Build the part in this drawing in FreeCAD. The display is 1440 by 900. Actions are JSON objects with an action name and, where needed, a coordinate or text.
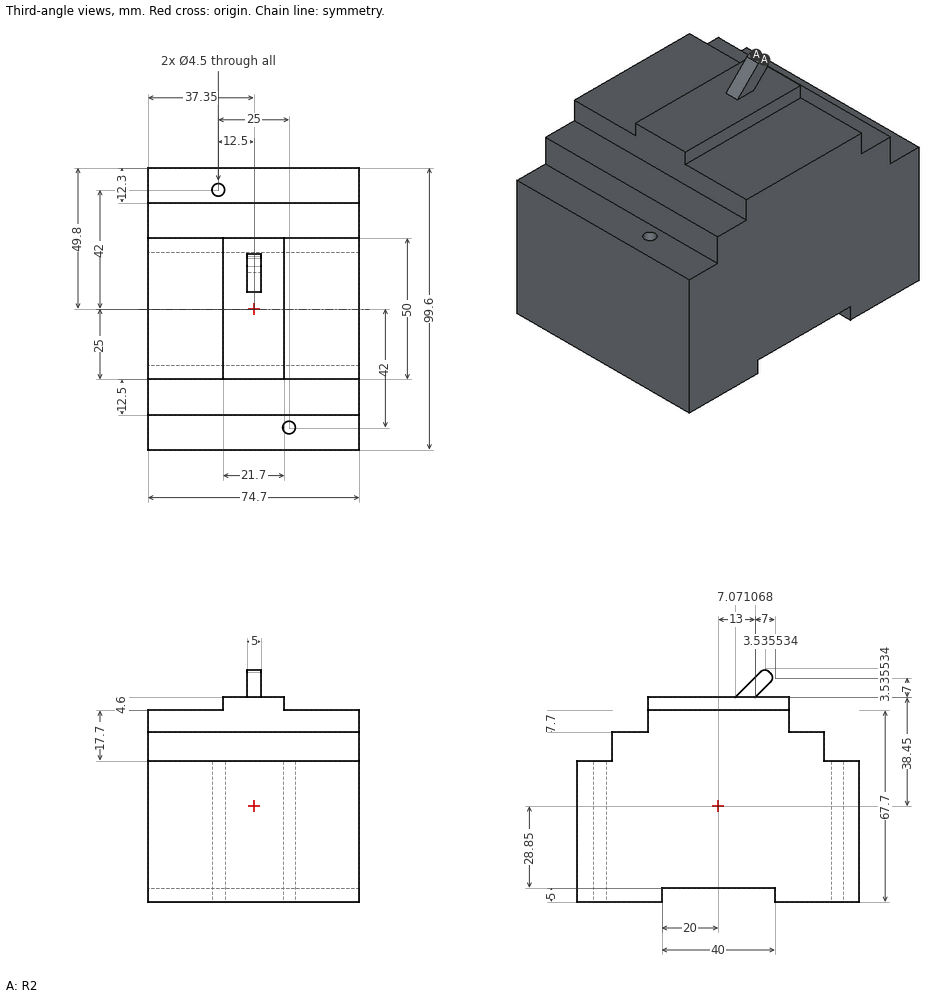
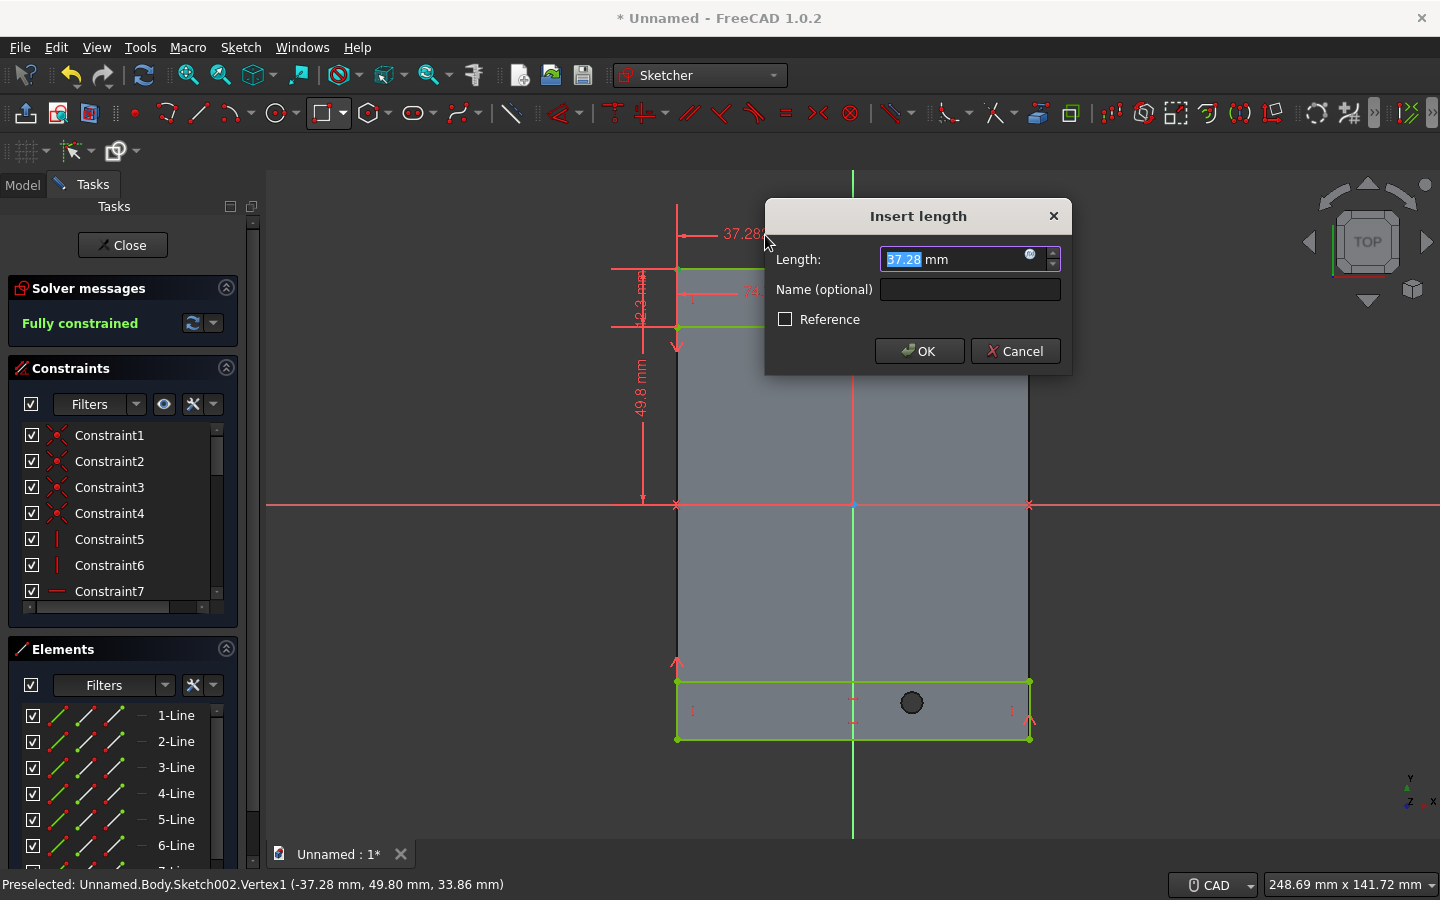
{"action": "type", "text": "37.35"}
{"action": "key", "text": "Return"}
{"action": "key", "text": "Escape"}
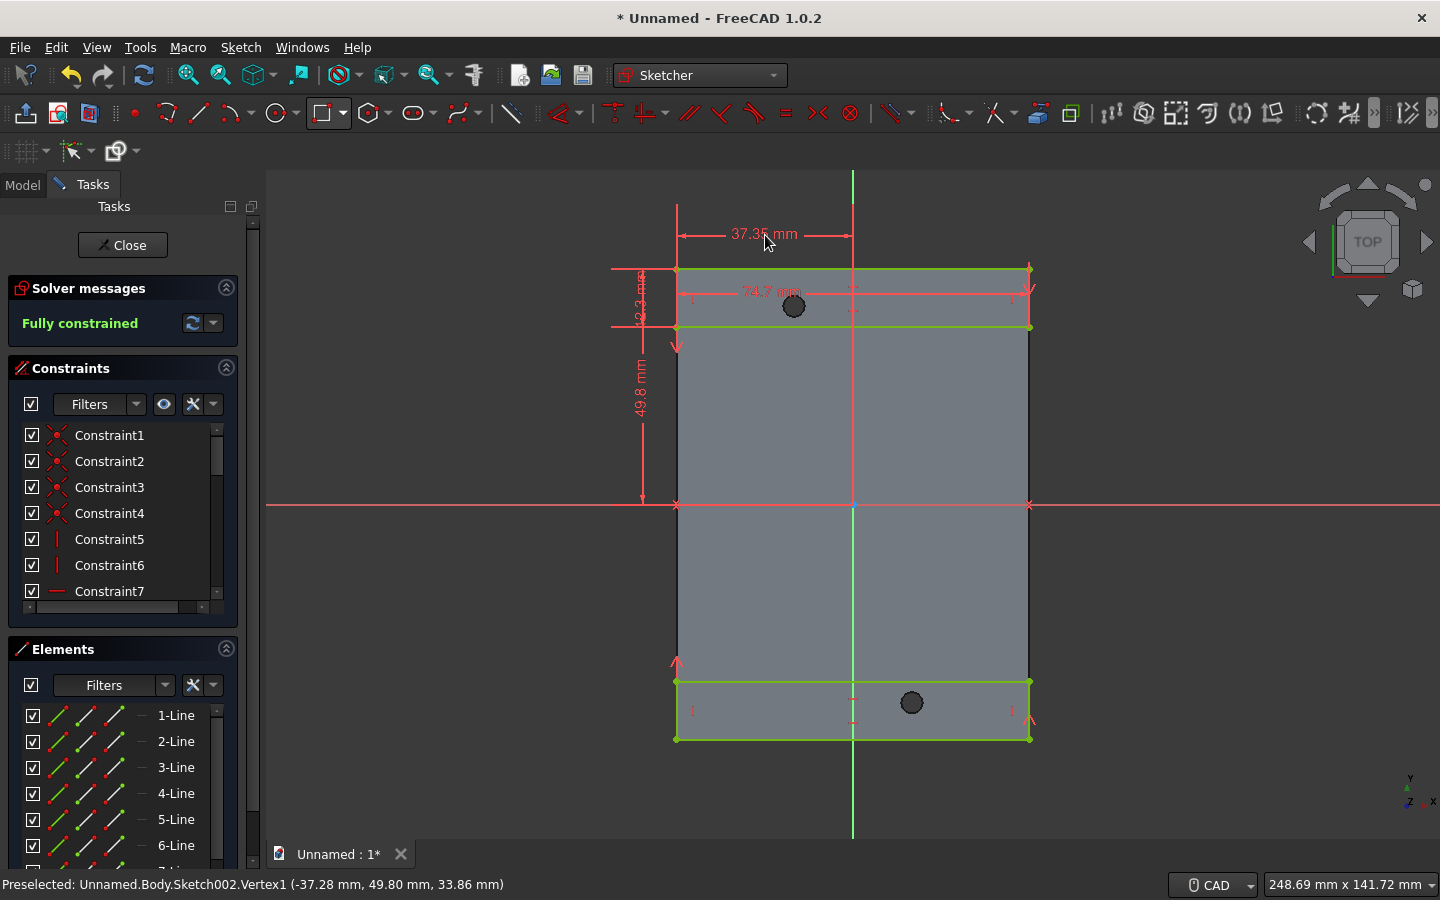
{"action": "left_click", "coordinate": [123, 245]}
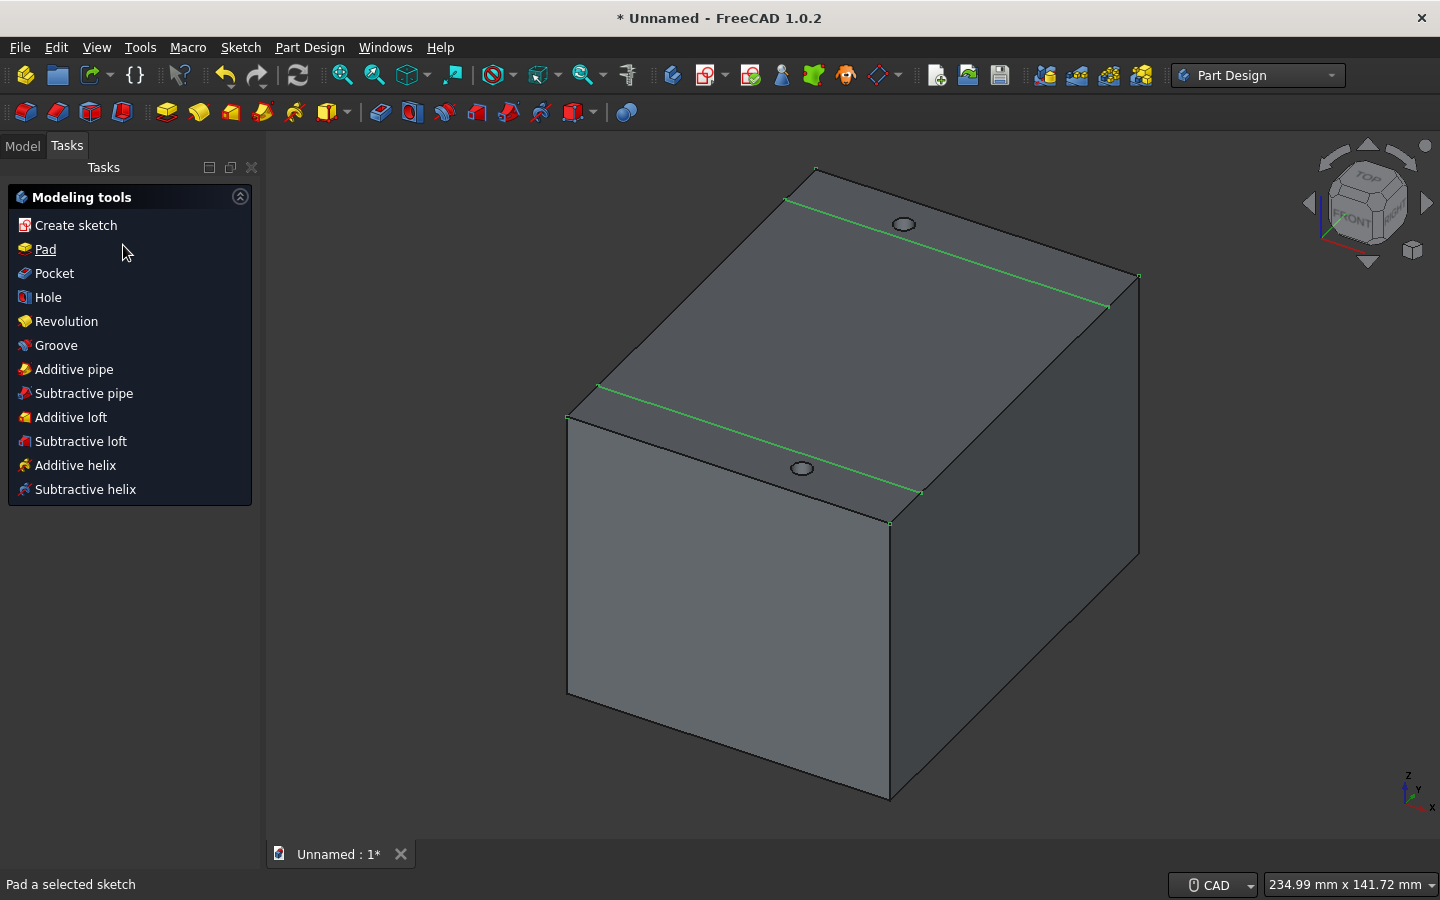
{"action": "left_click", "coordinate": [382, 112]}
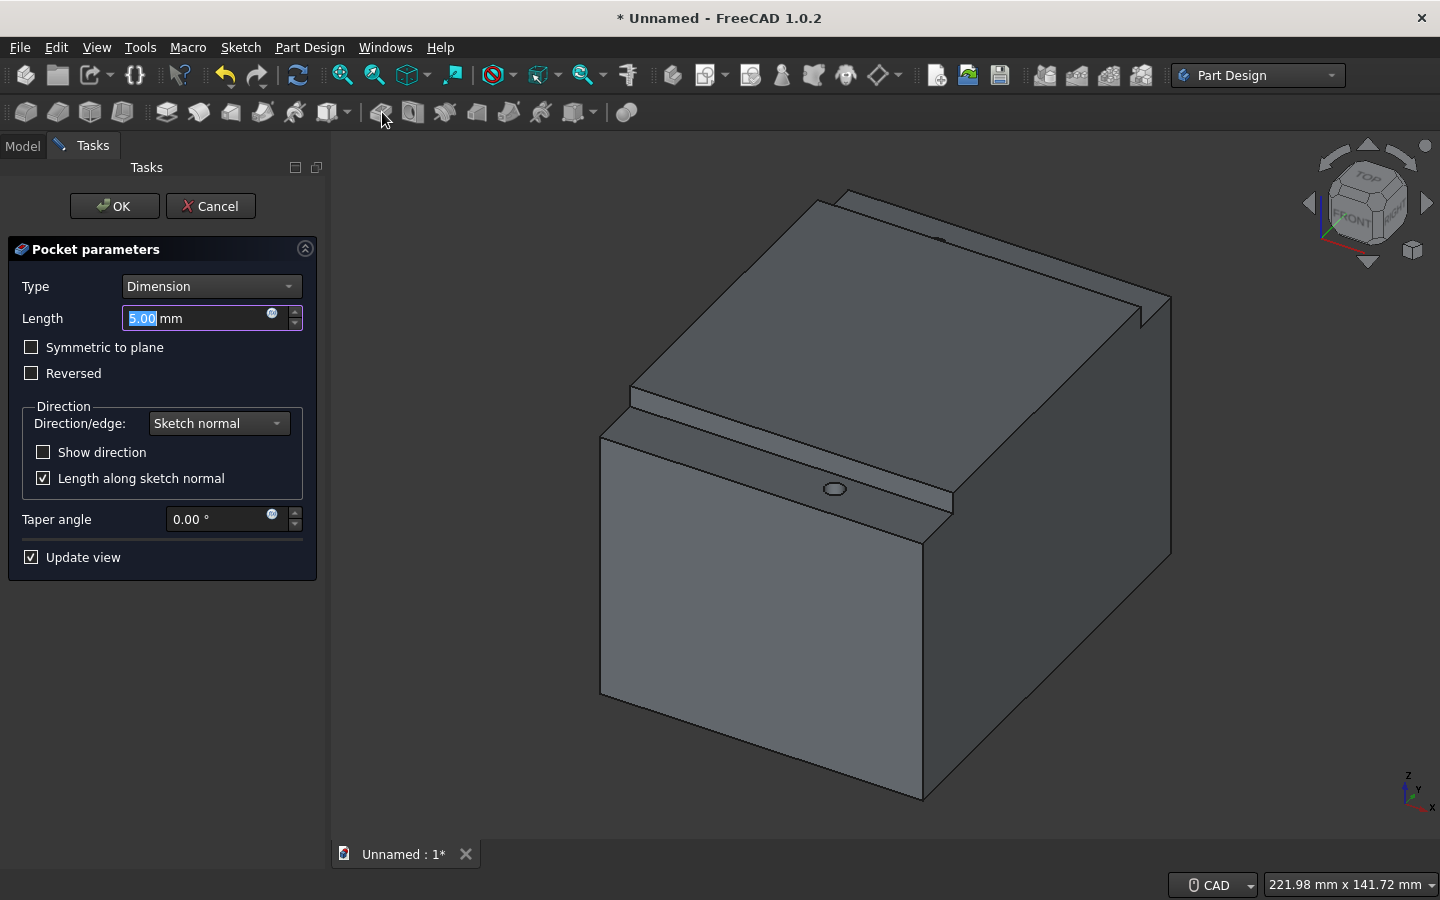
{"action": "type", "text": "17.7"}
{"action": "key", "text": "Tab"}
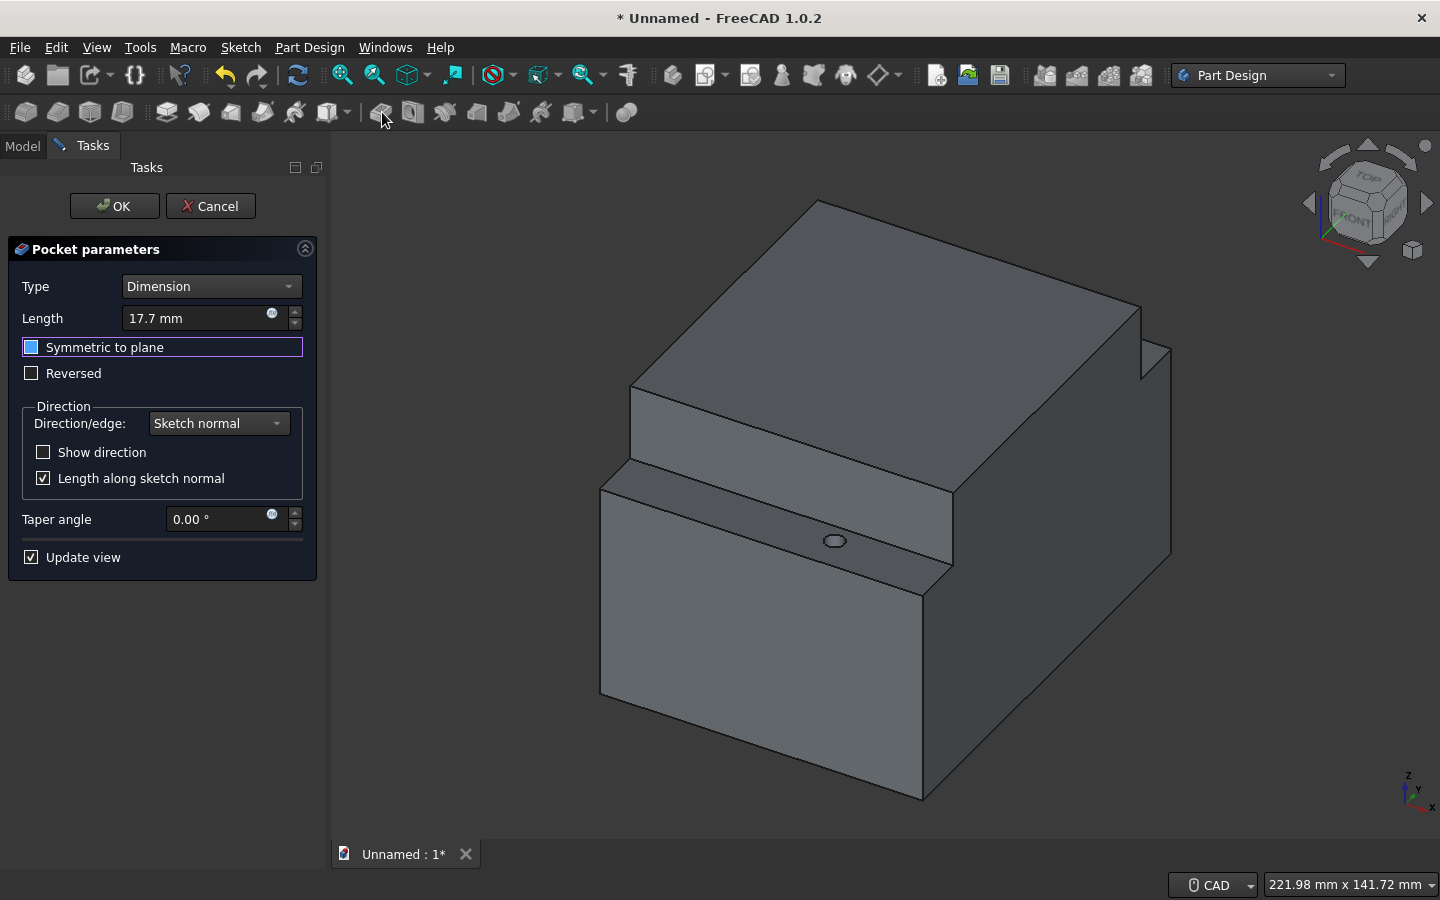
{"action": "left_click", "coordinate": [115, 206]}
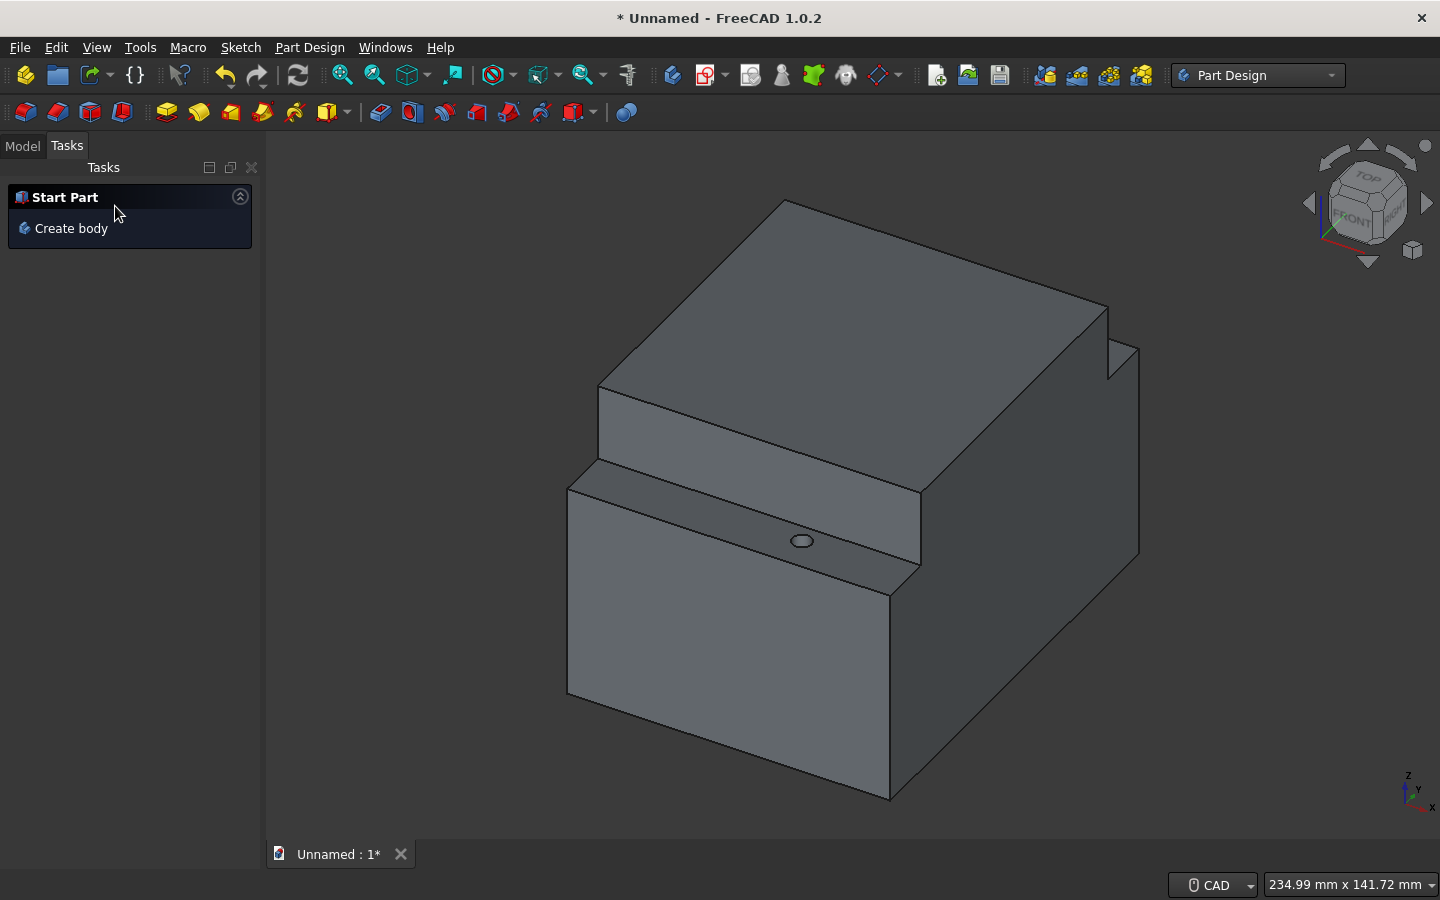
{"action": "left_click", "coordinate": [853, 345]}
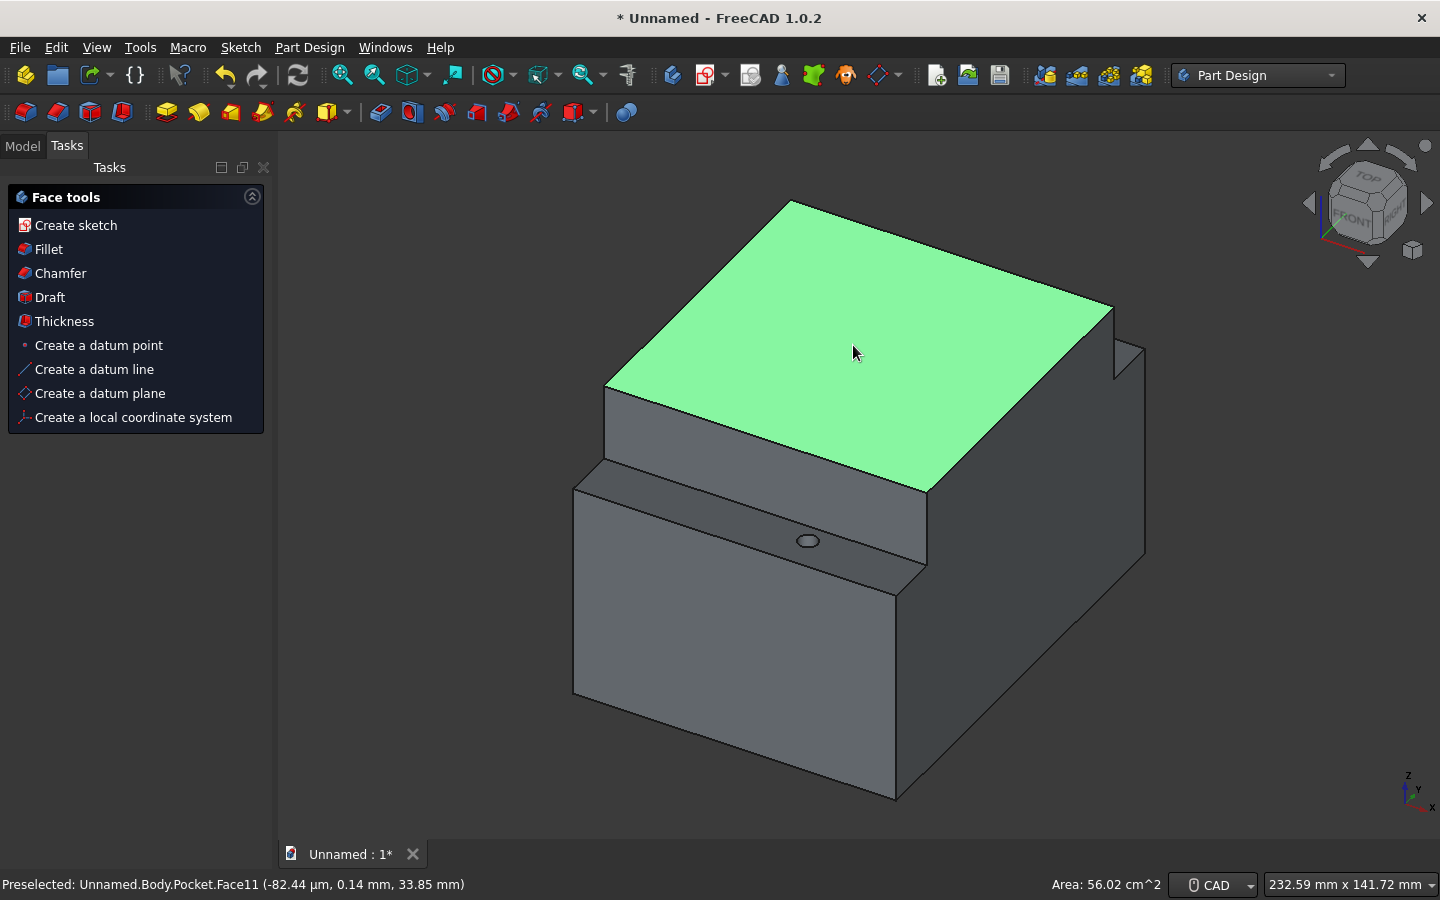
{"action": "left_click", "coordinate": [706, 76]}